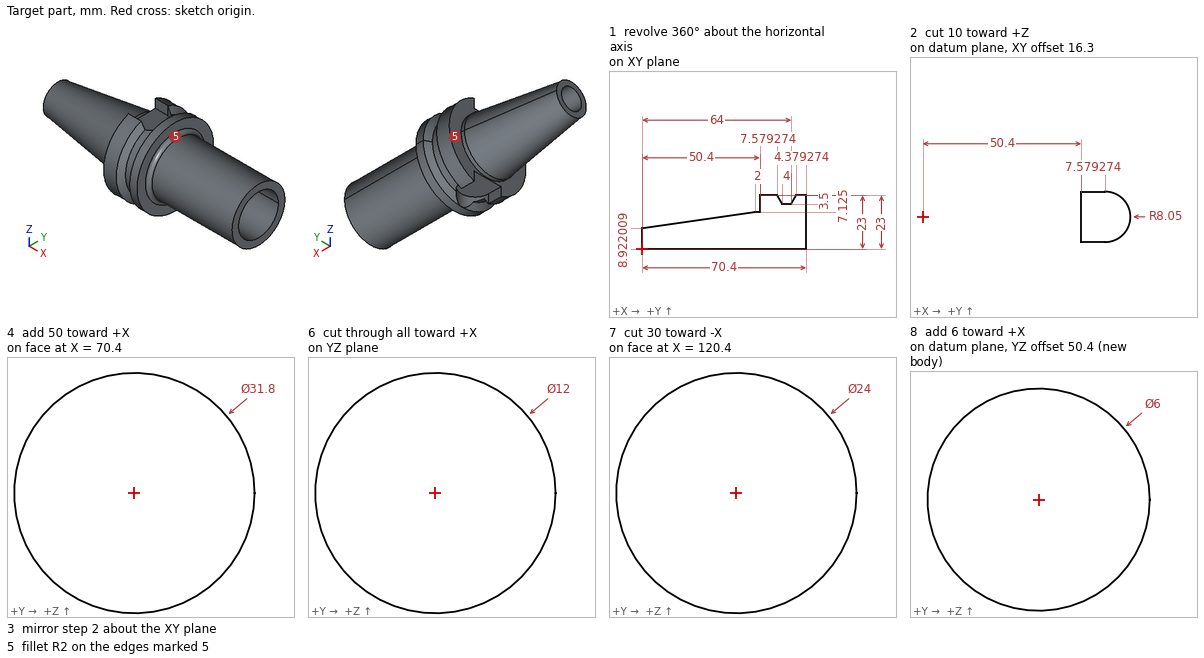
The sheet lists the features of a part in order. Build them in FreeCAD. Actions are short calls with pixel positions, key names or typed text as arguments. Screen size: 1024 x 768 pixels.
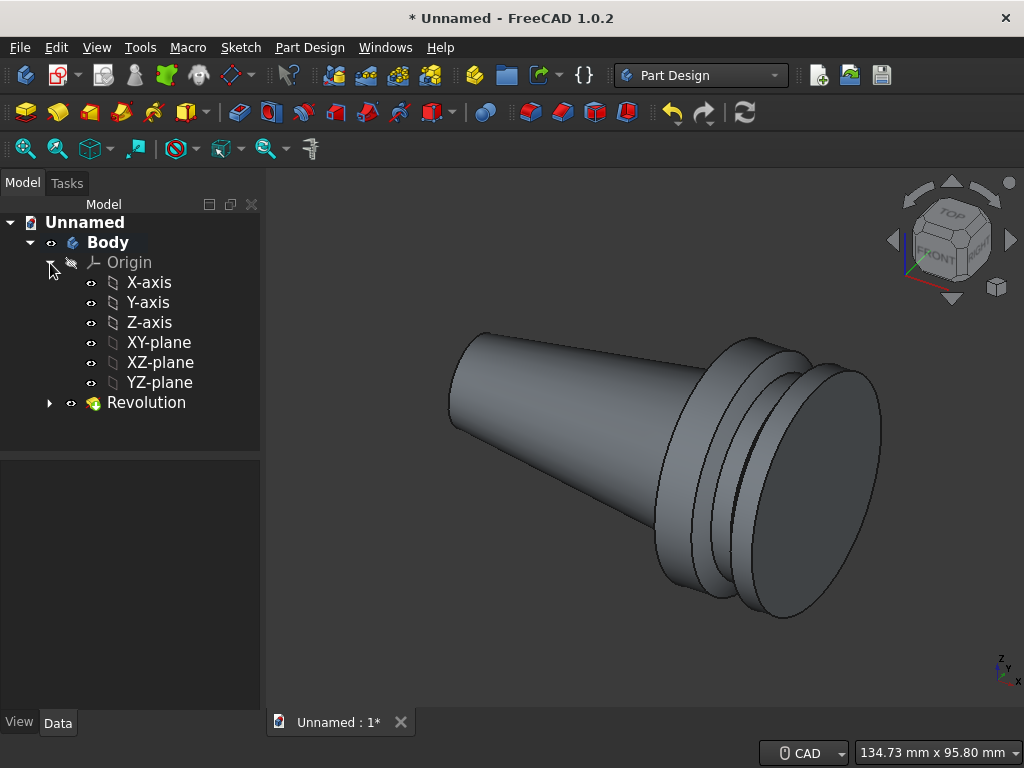
click(136, 343)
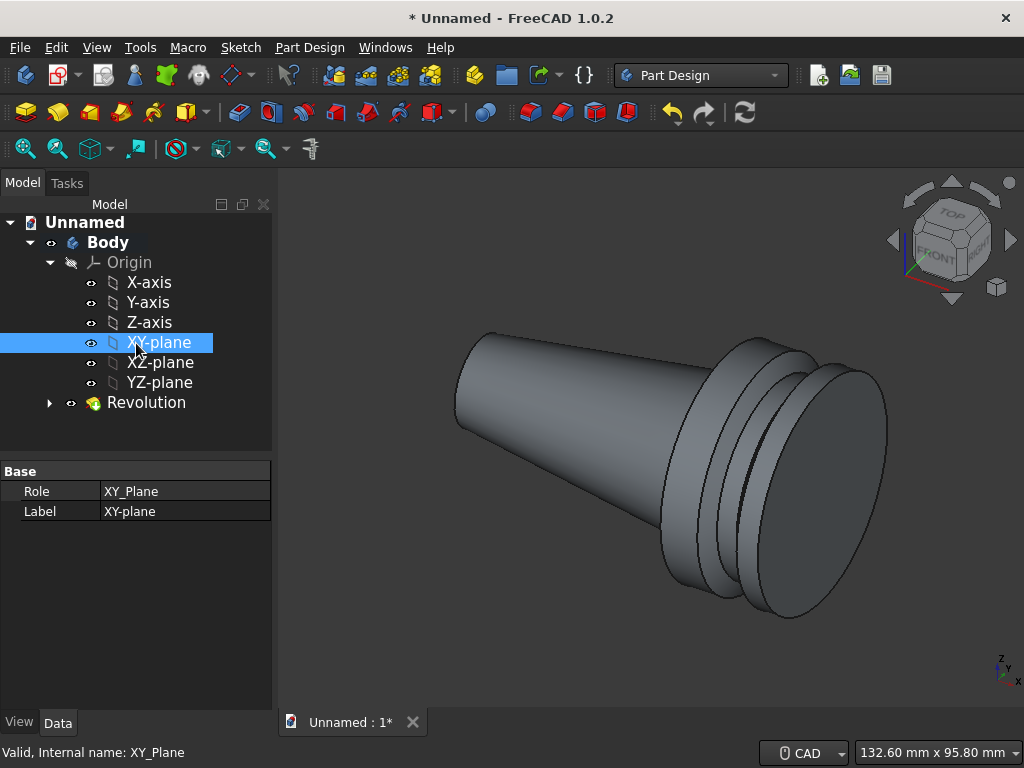
click(232, 76)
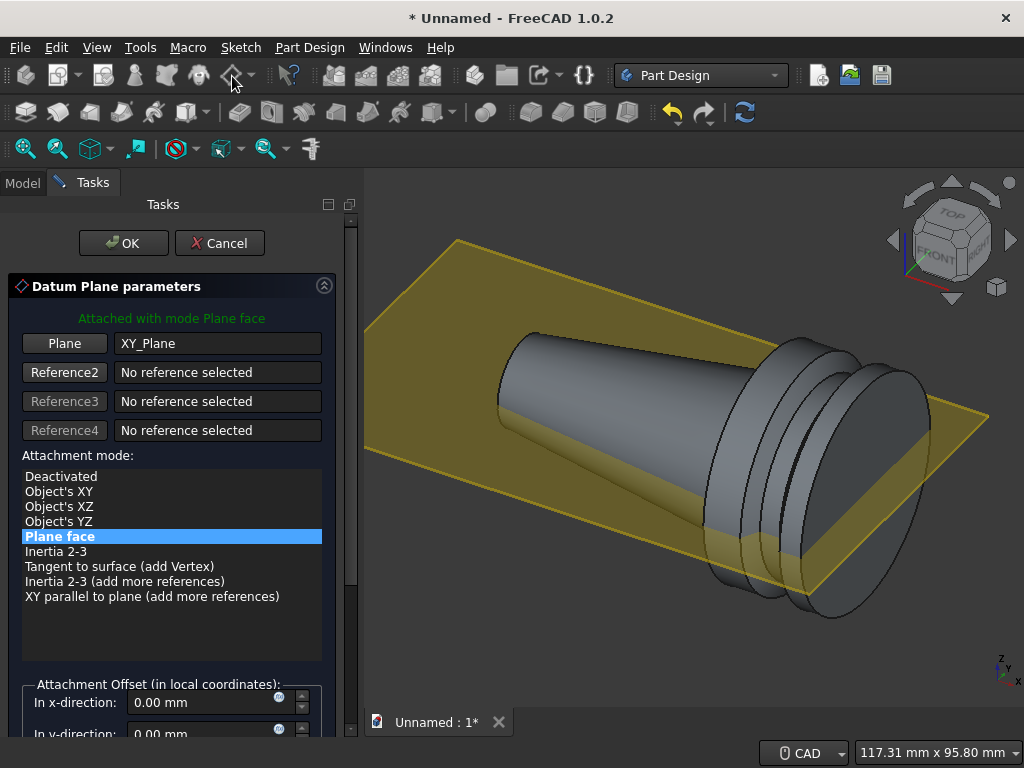
scroll(351, 475, down, 2)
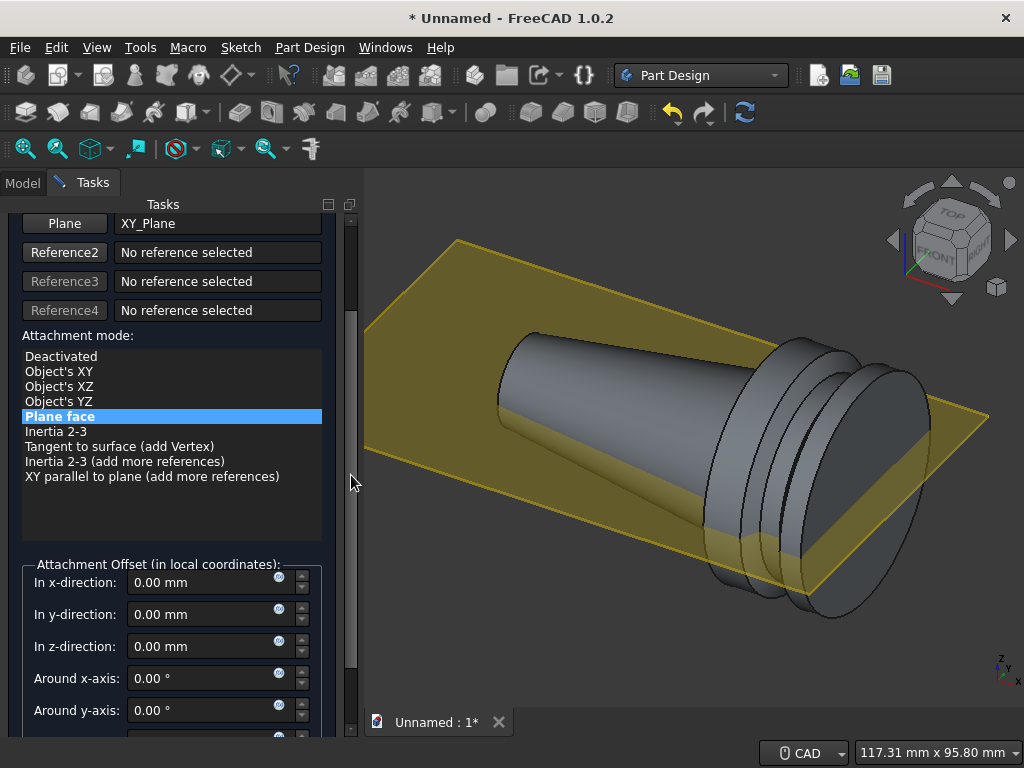
triple_click(210, 646)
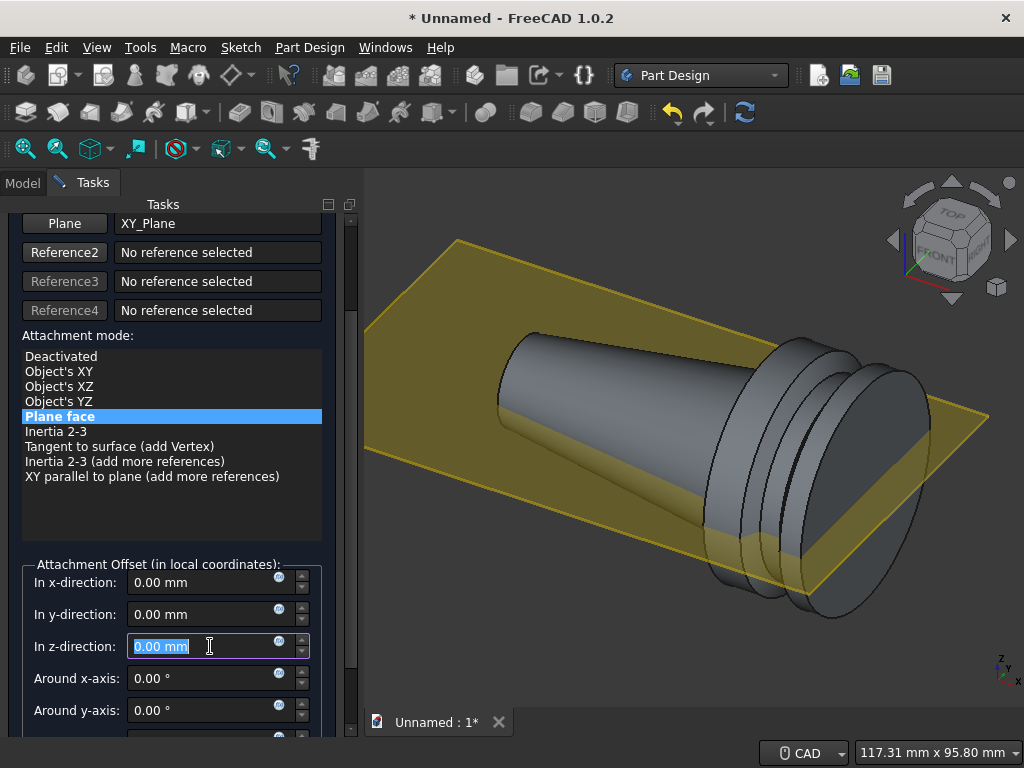
text(16.3)
key(Tab)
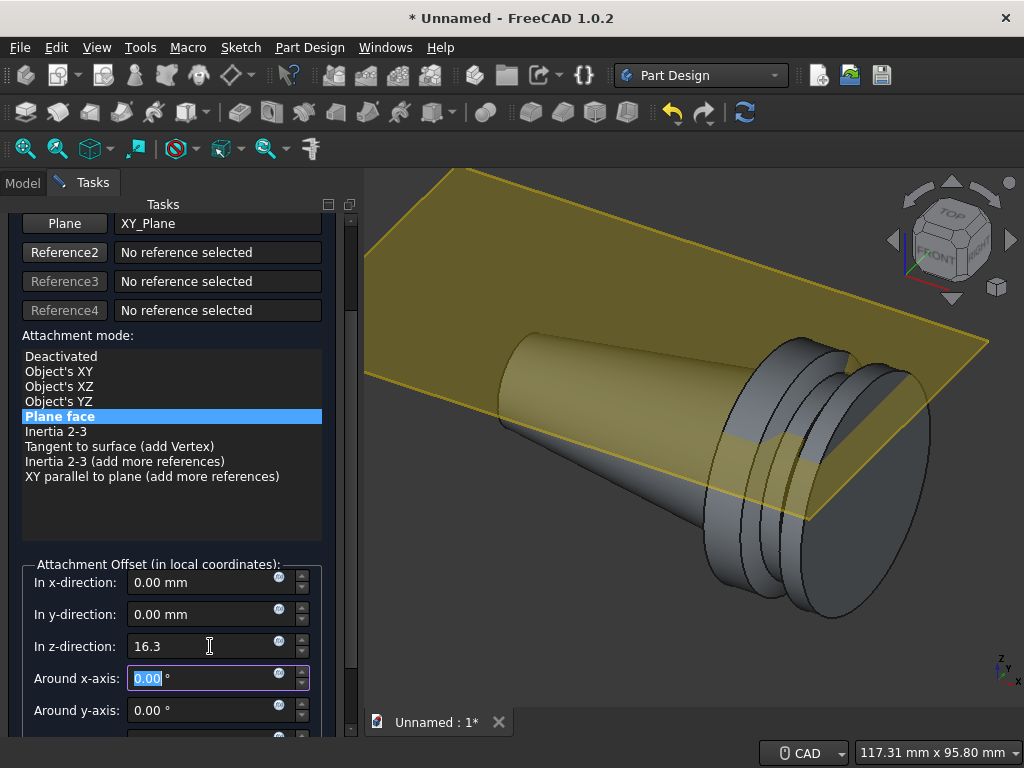
scroll(351, 475, up, 3)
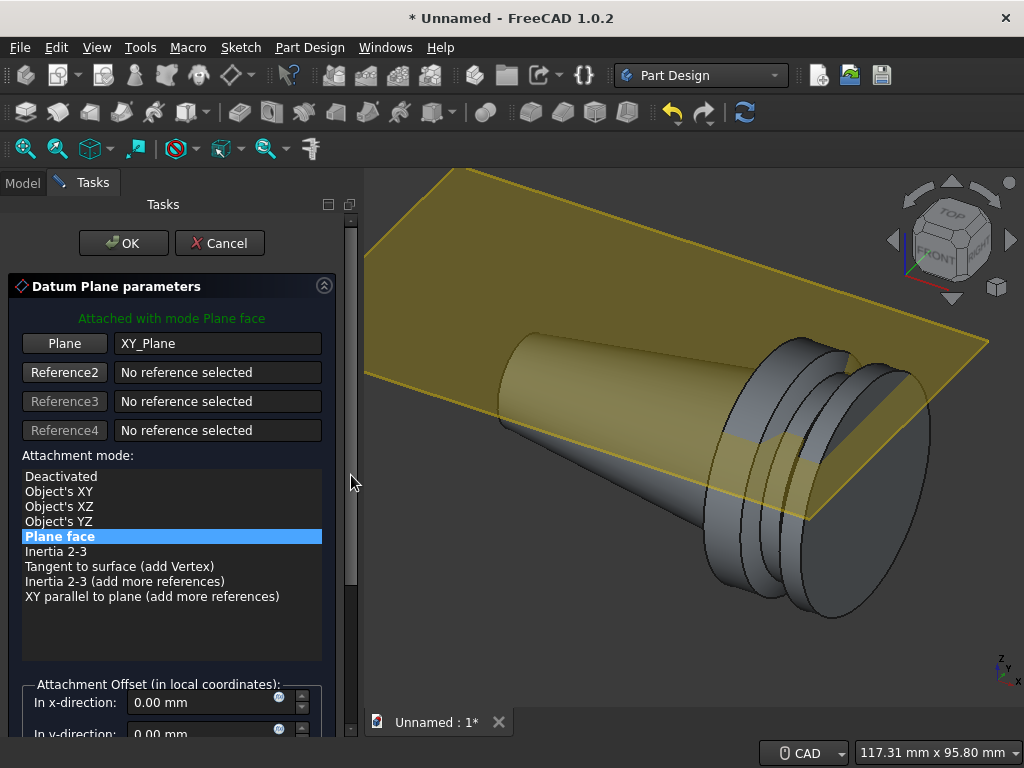
click(124, 243)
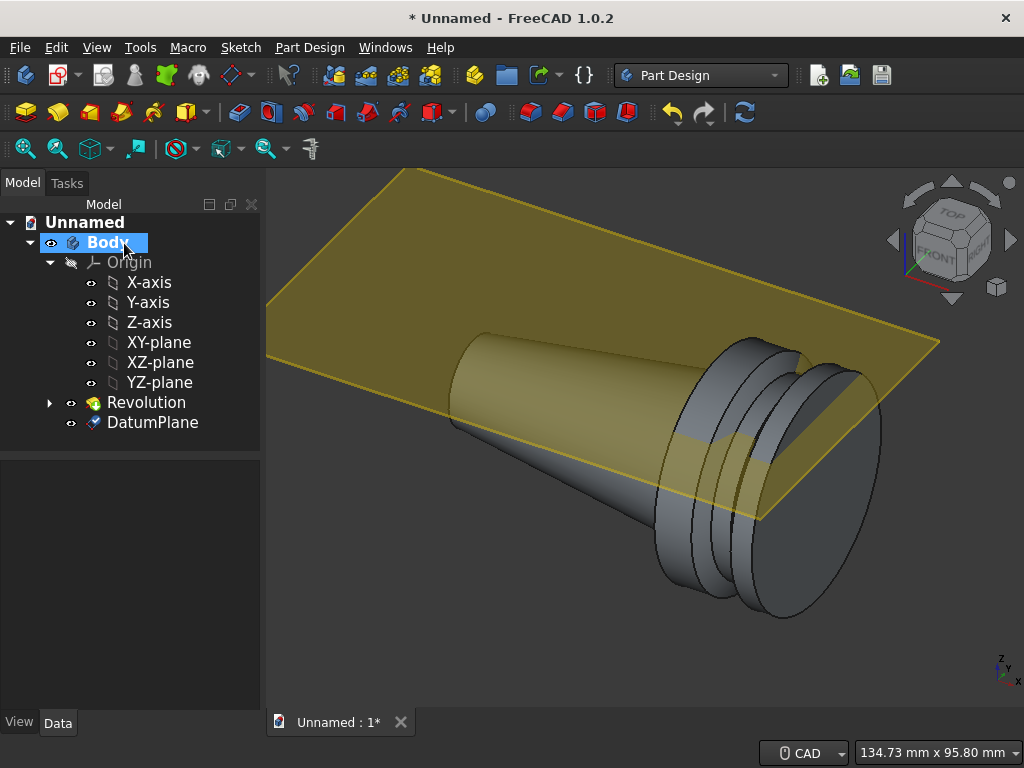
click(116, 423)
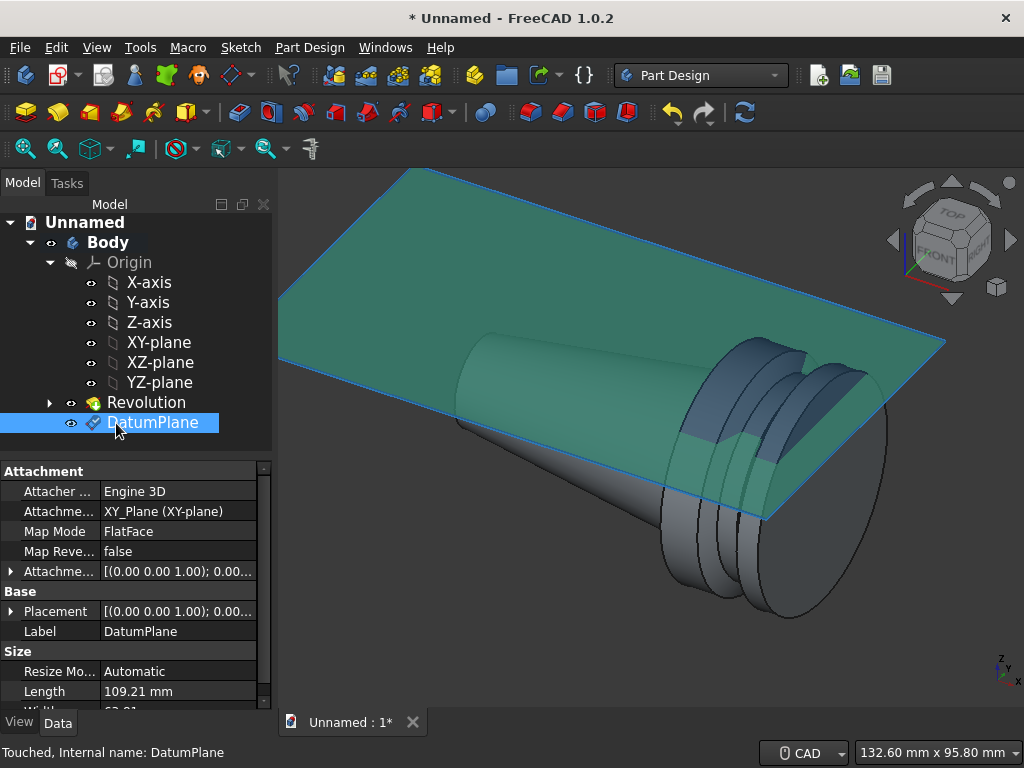
click(58, 76)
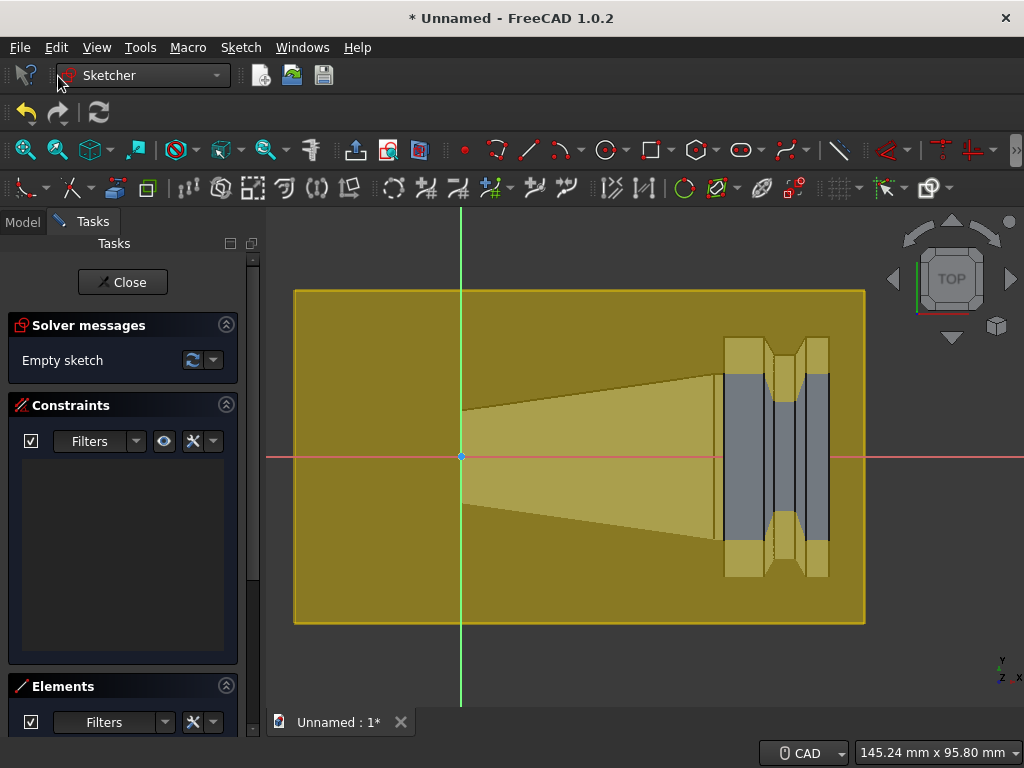
click(420, 150)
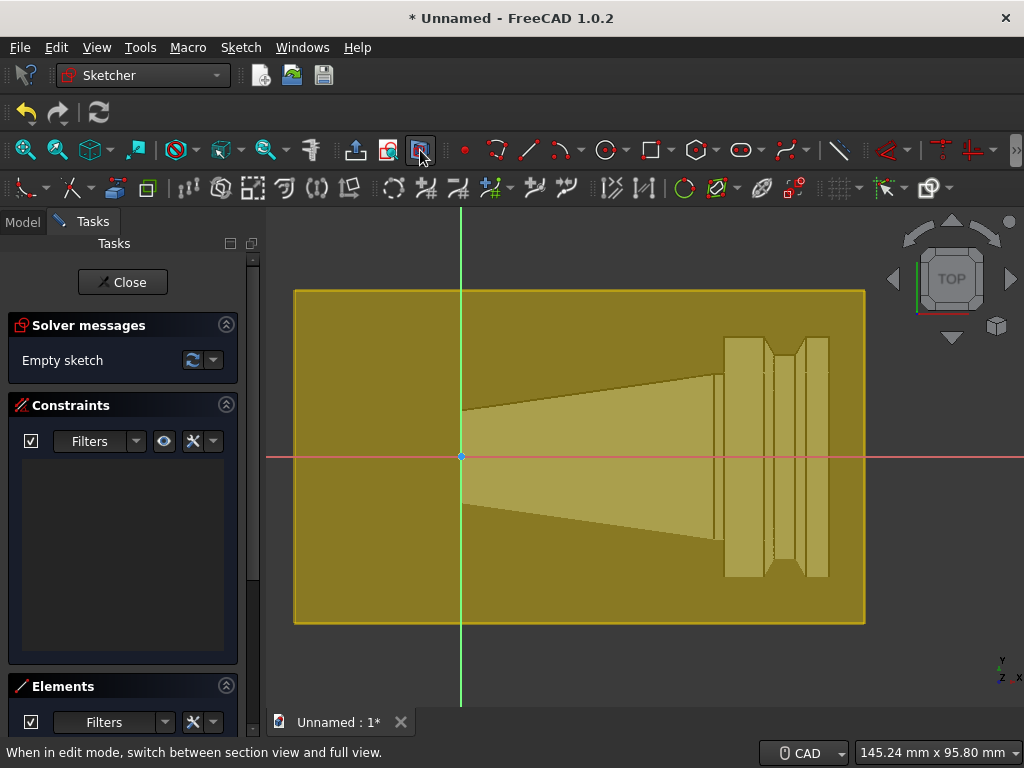
scroll(827, 457, up, 7)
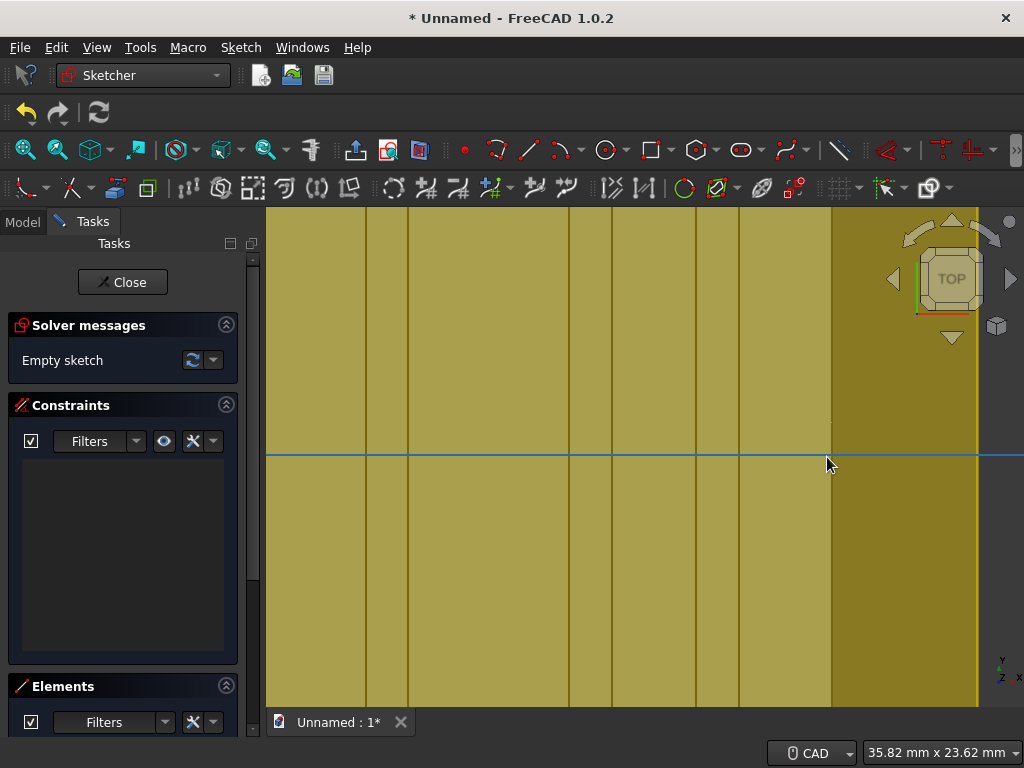
click(498, 150)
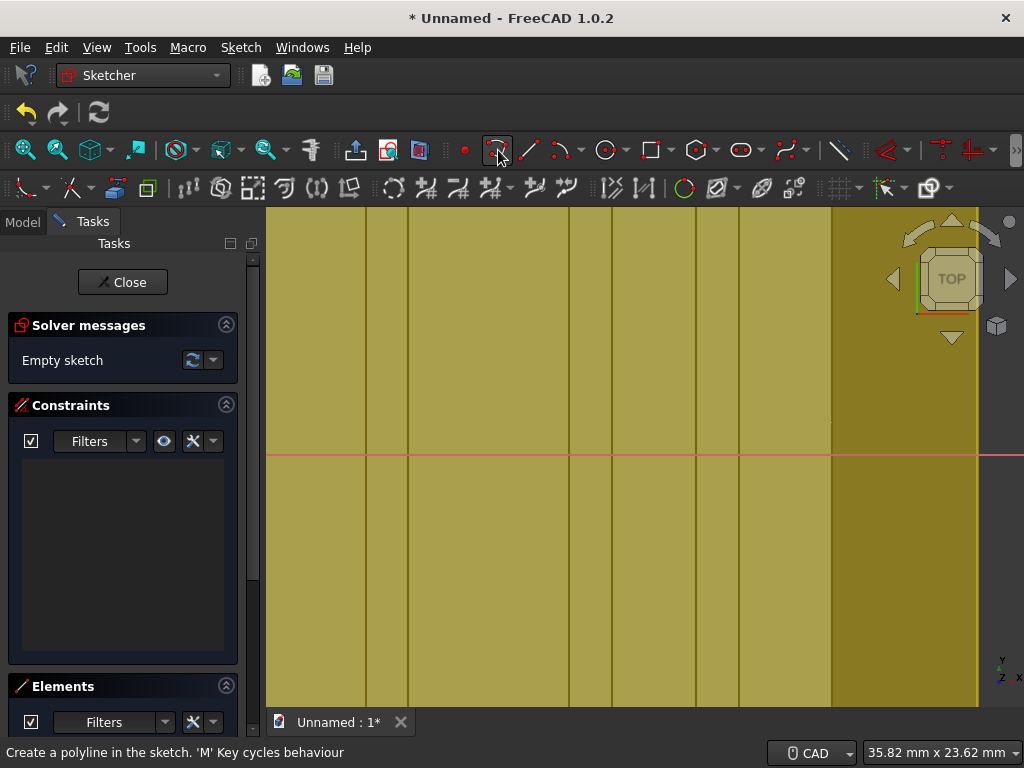
click(569, 285)
click(408, 285)
click(408, 626)
click(569, 626)
right_click(569, 626)